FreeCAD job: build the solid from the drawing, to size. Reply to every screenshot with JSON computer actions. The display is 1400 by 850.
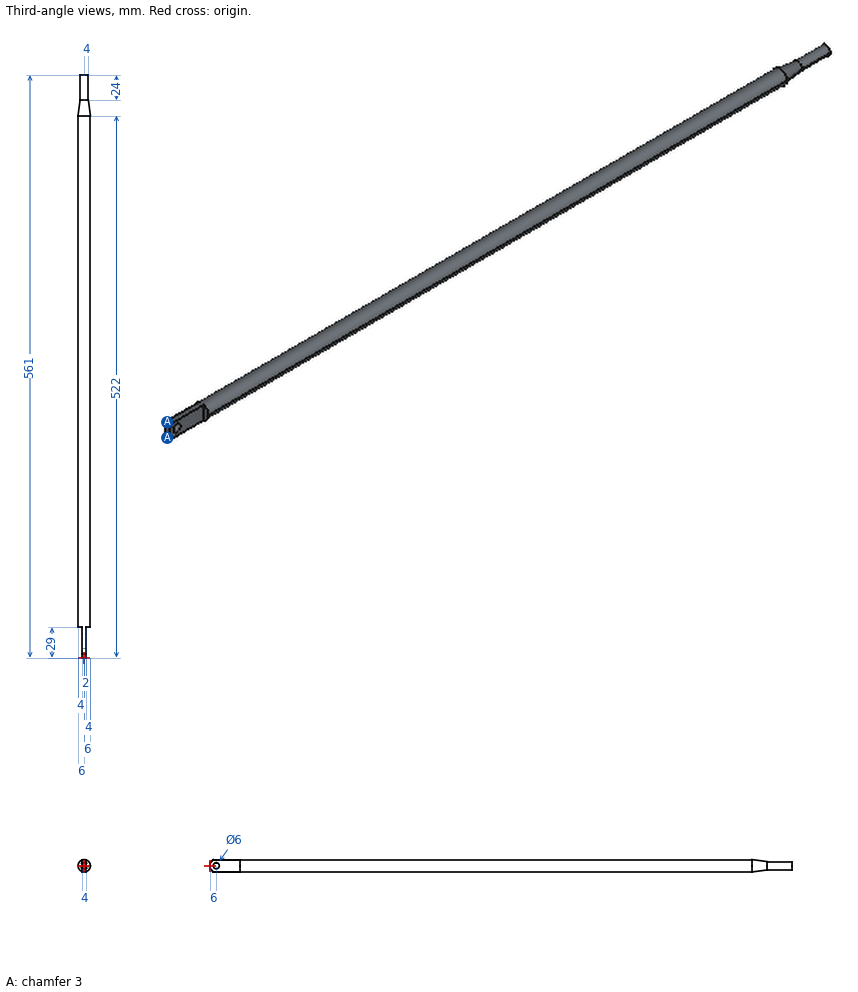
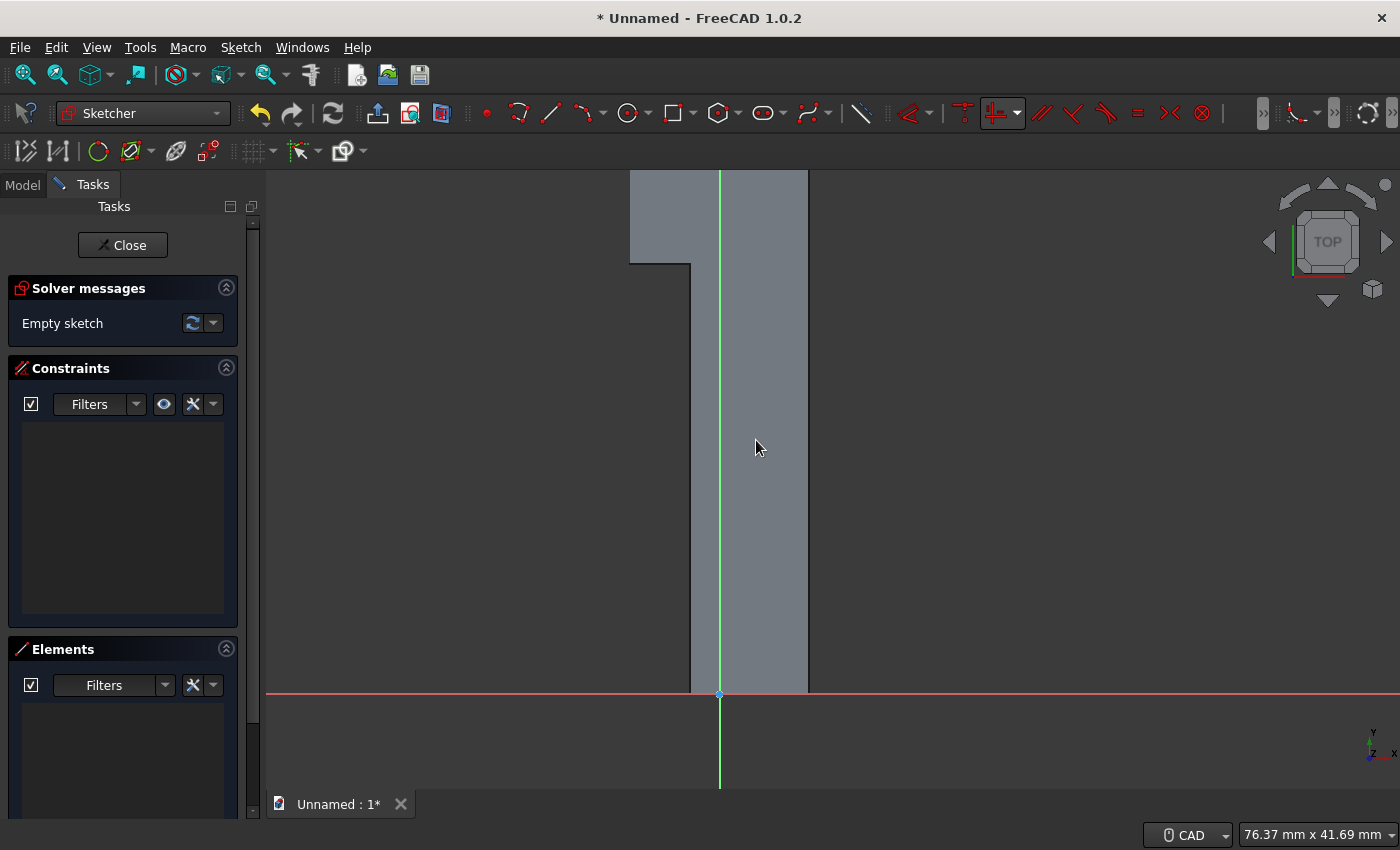
{"action": "left_click", "coordinate": [674, 114]}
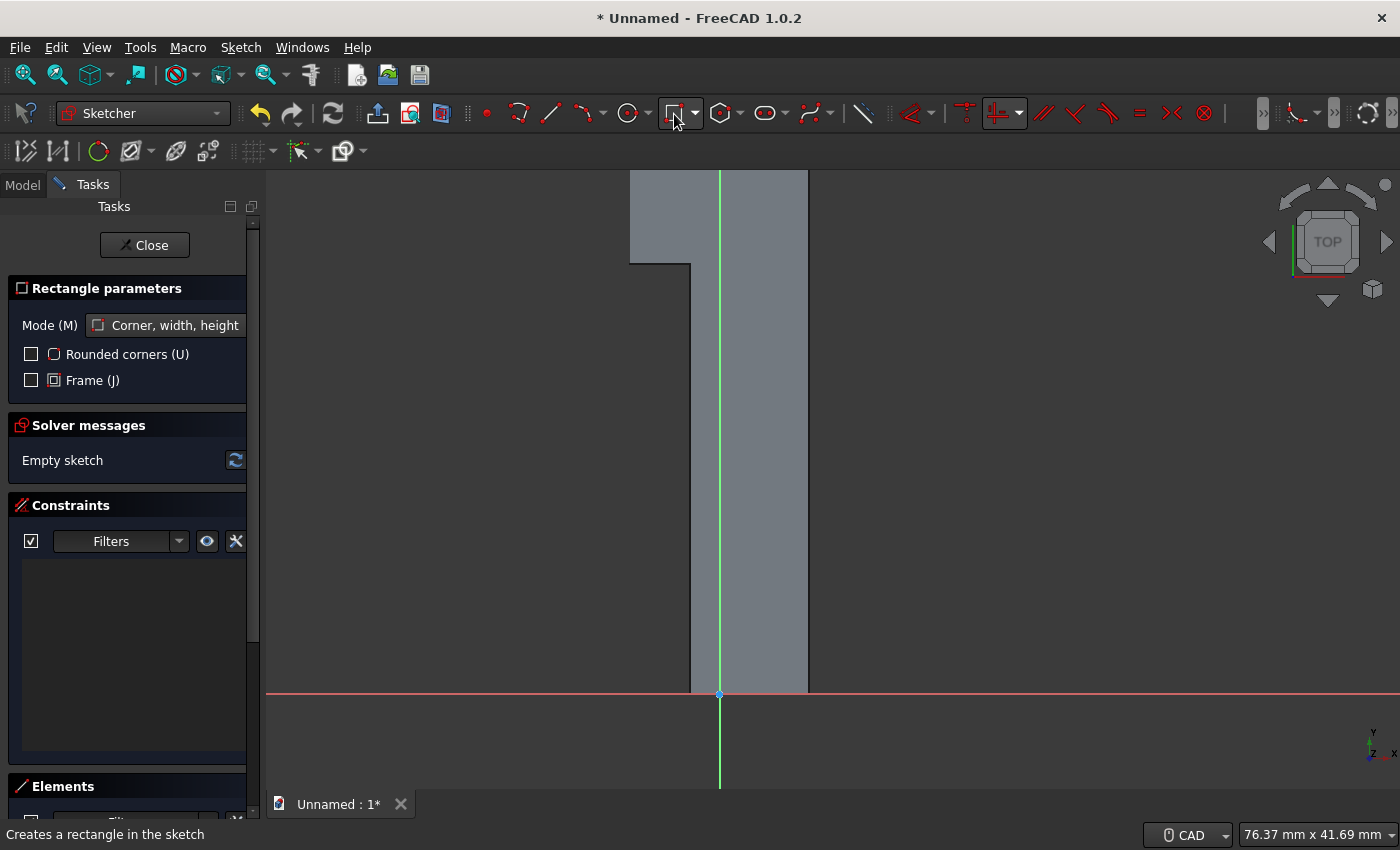
{"action": "left_click", "coordinate": [749, 264]}
{"action": "left_click", "coordinate": [809, 694]}
{"action": "key", "text": "Escape"}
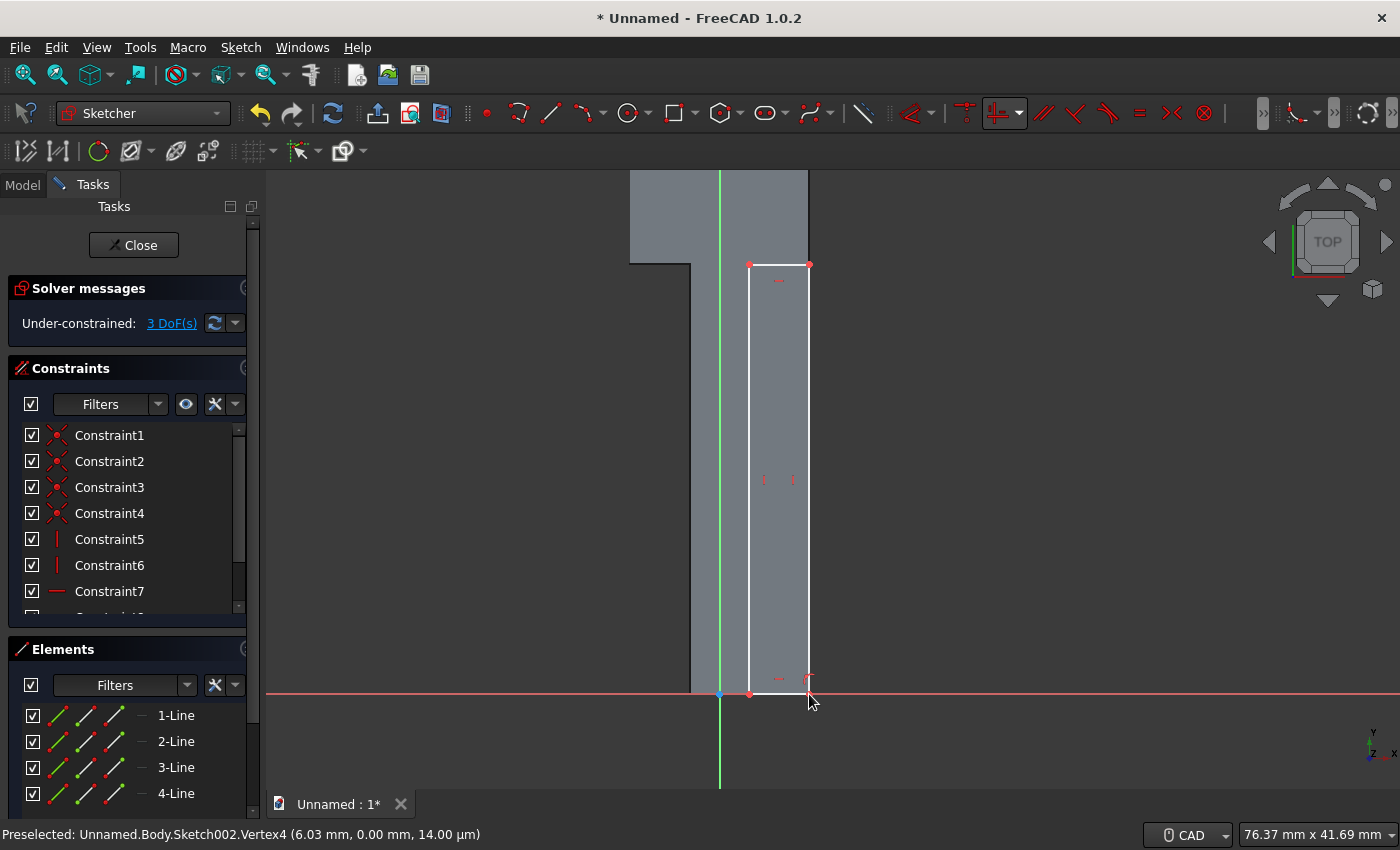
{"action": "left_click", "coordinate": [910, 114]}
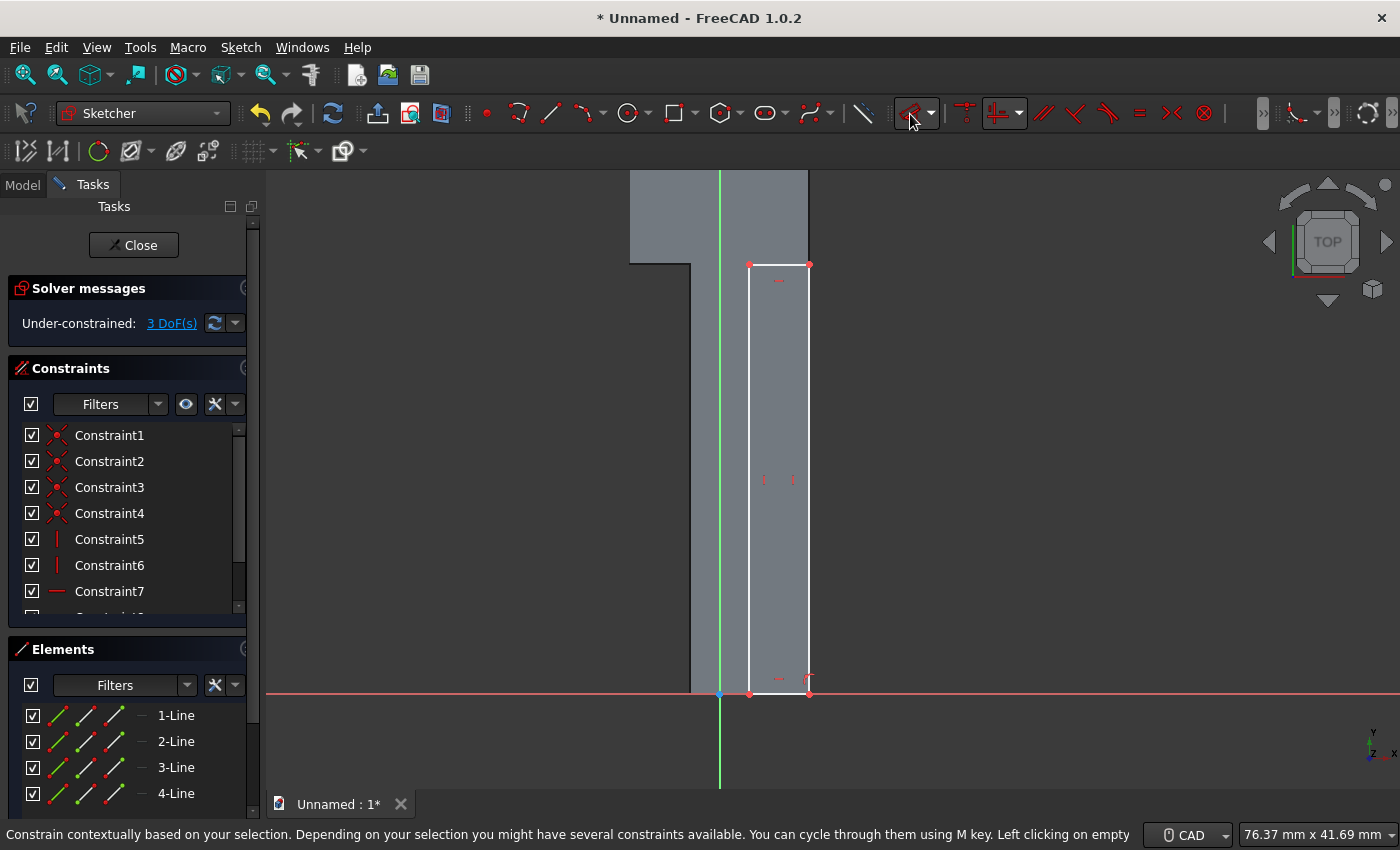
{"action": "left_click", "coordinate": [767, 694]}
{"action": "left_click", "coordinate": [779, 728]}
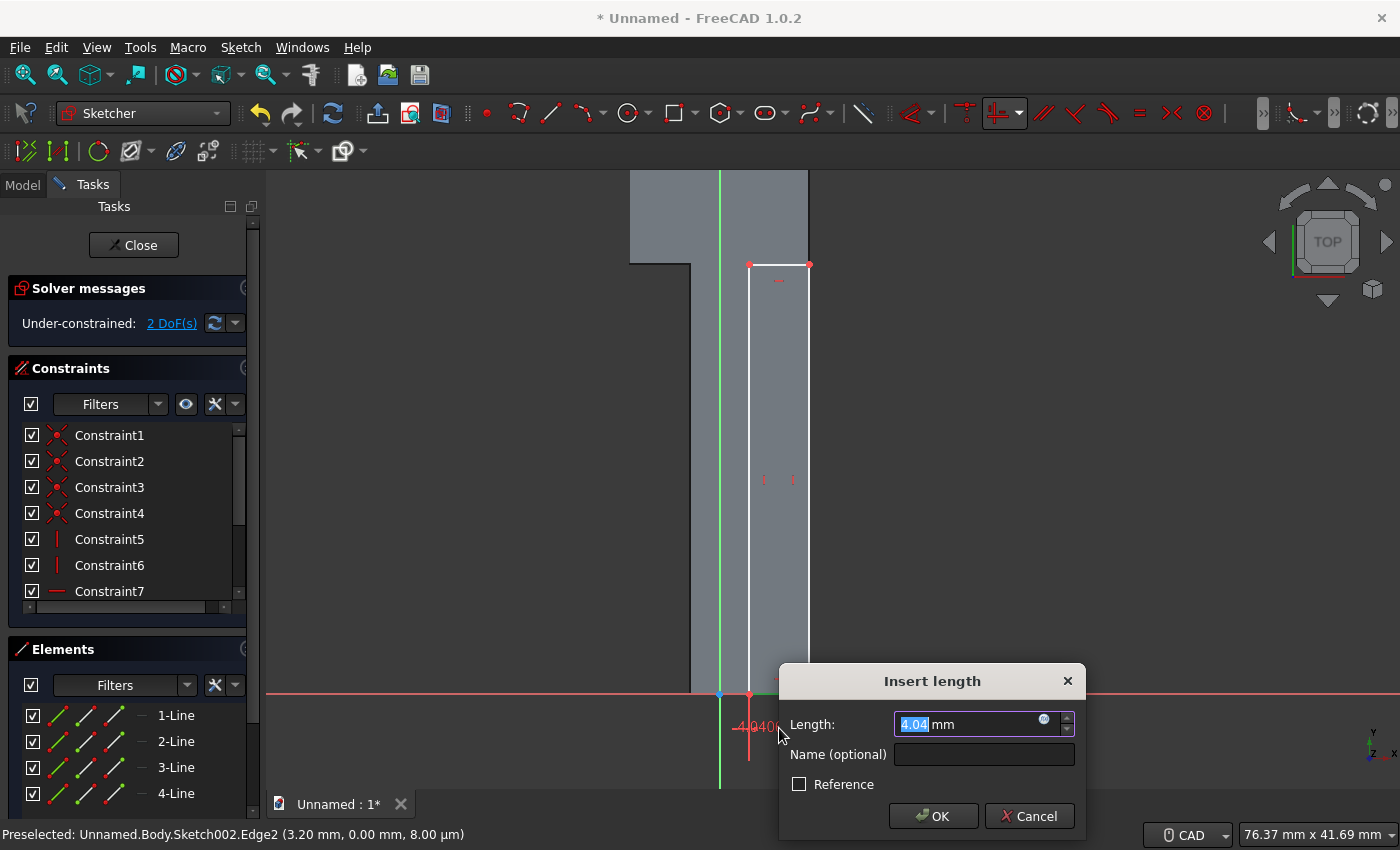
{"action": "type", "text": "4"}
{"action": "key", "text": "Return"}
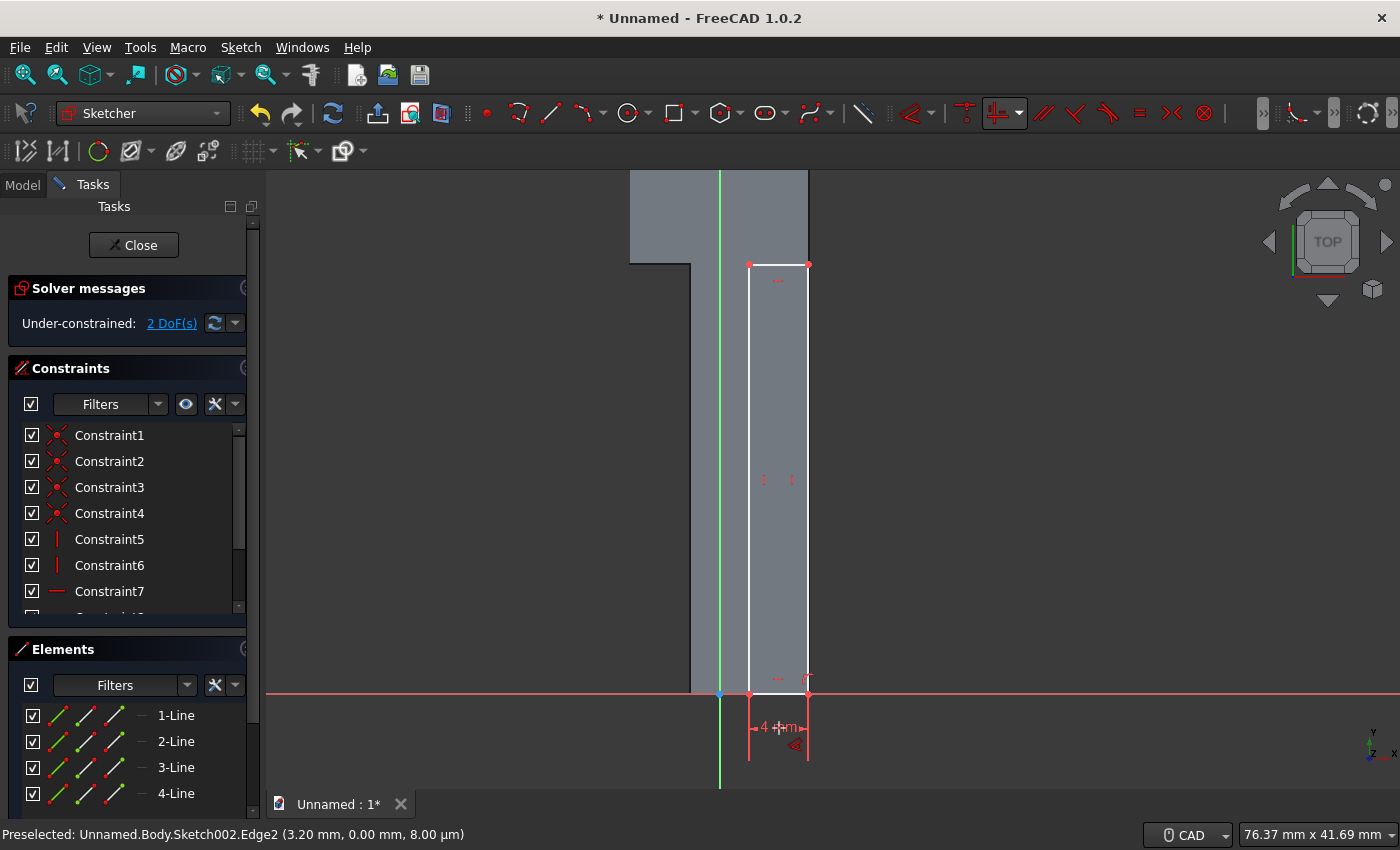
{"action": "left_click", "coordinate": [749, 394]}
{"action": "left_click", "coordinate": [783, 480]}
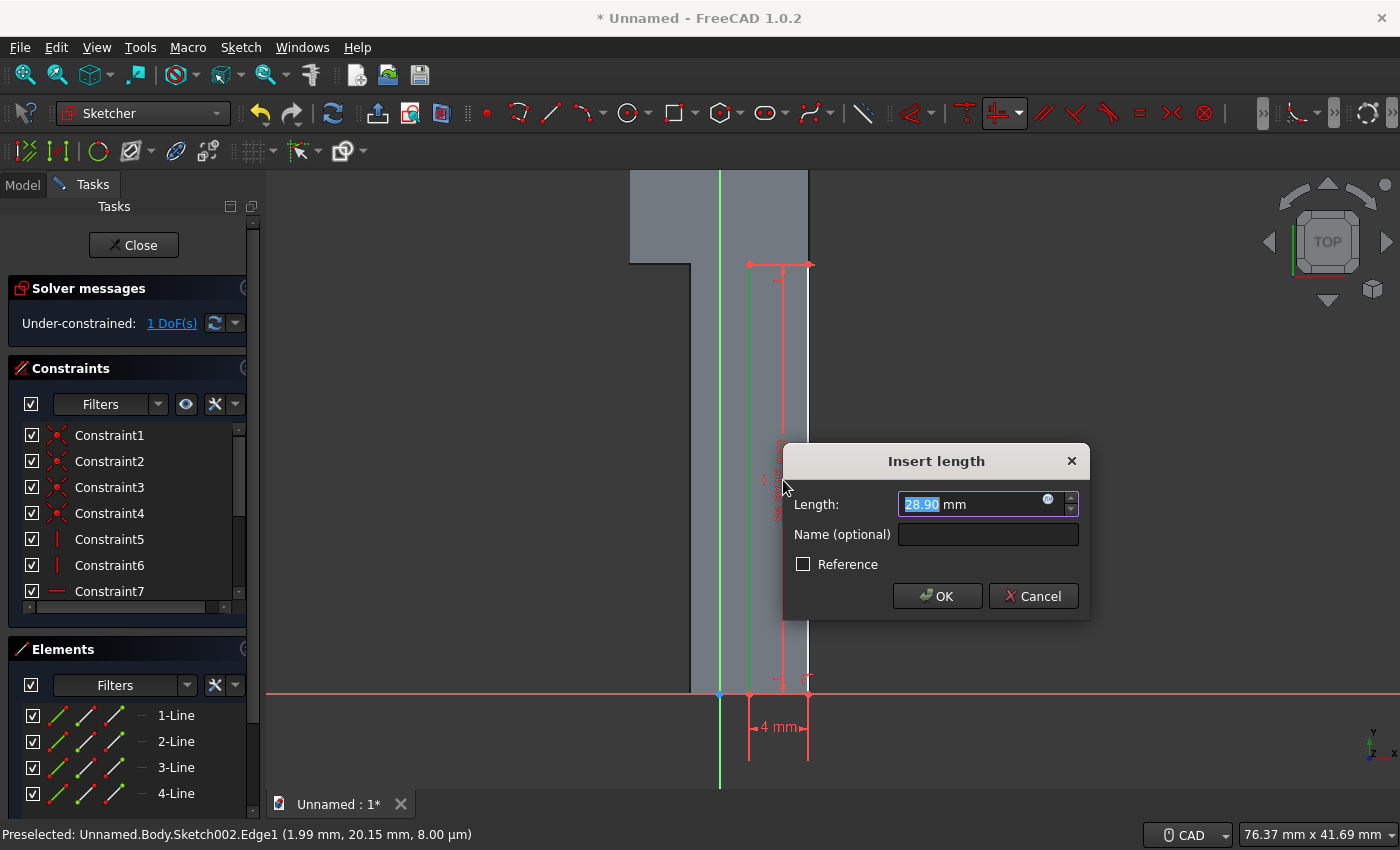
{"action": "type", "text": "29"}
{"action": "key", "text": "Return"}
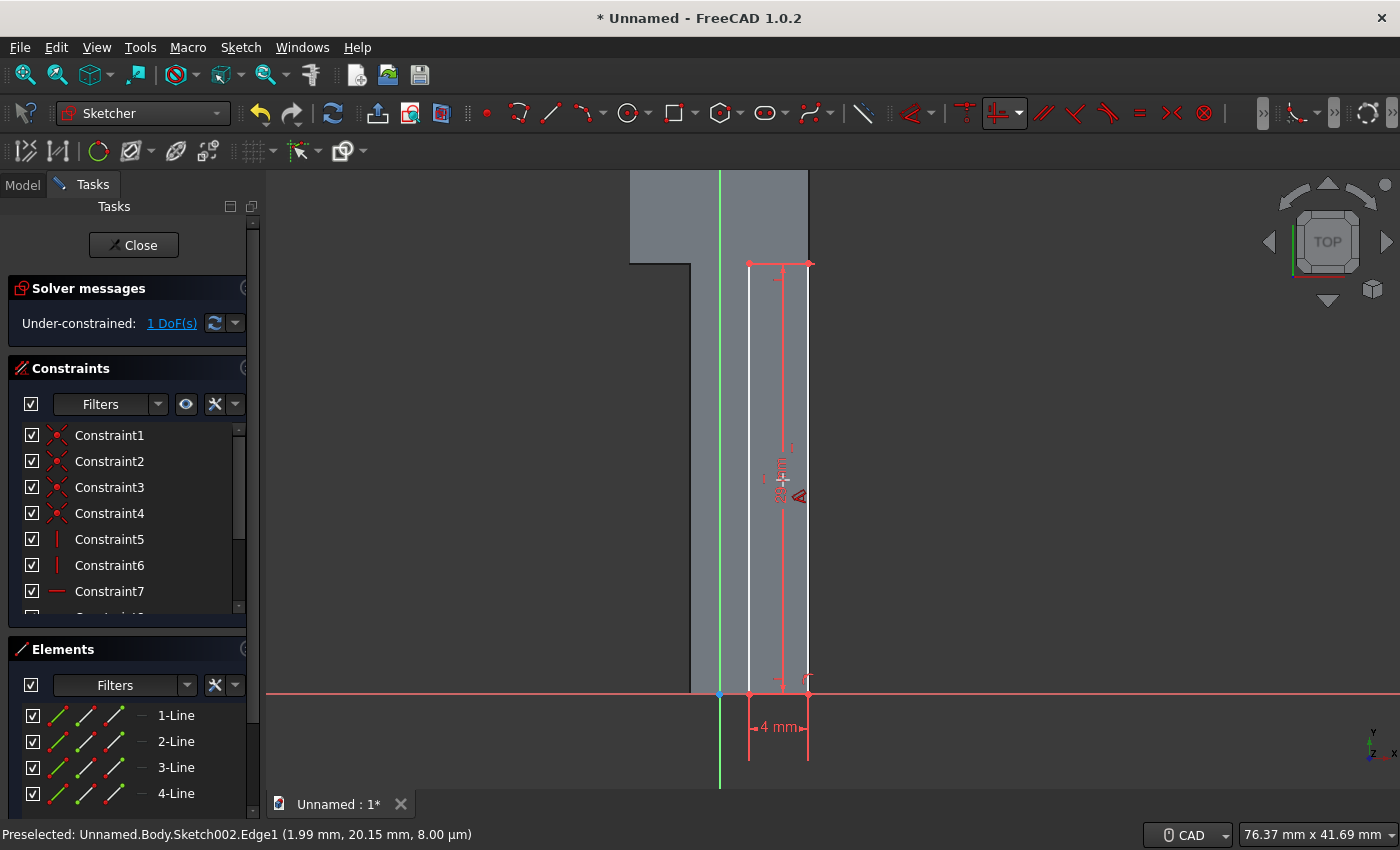
{"action": "scroll", "coordinate": [749, 264], "scroll_direction": "up", "scroll_amount": 2}